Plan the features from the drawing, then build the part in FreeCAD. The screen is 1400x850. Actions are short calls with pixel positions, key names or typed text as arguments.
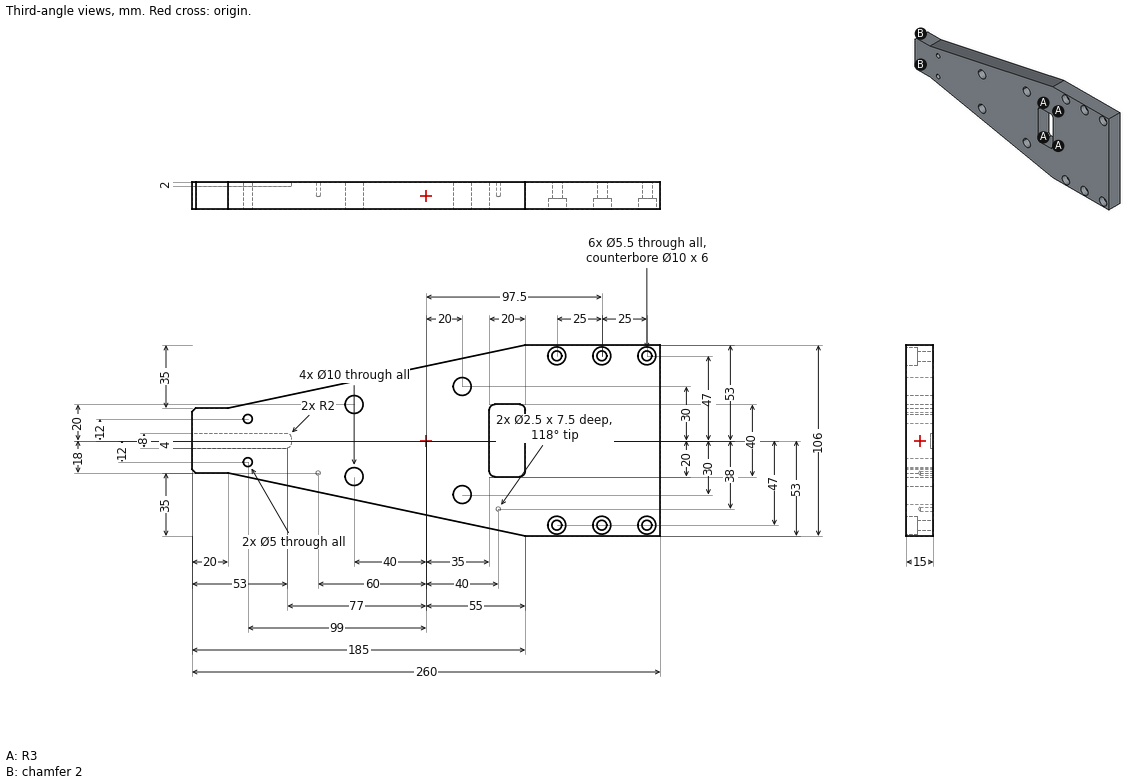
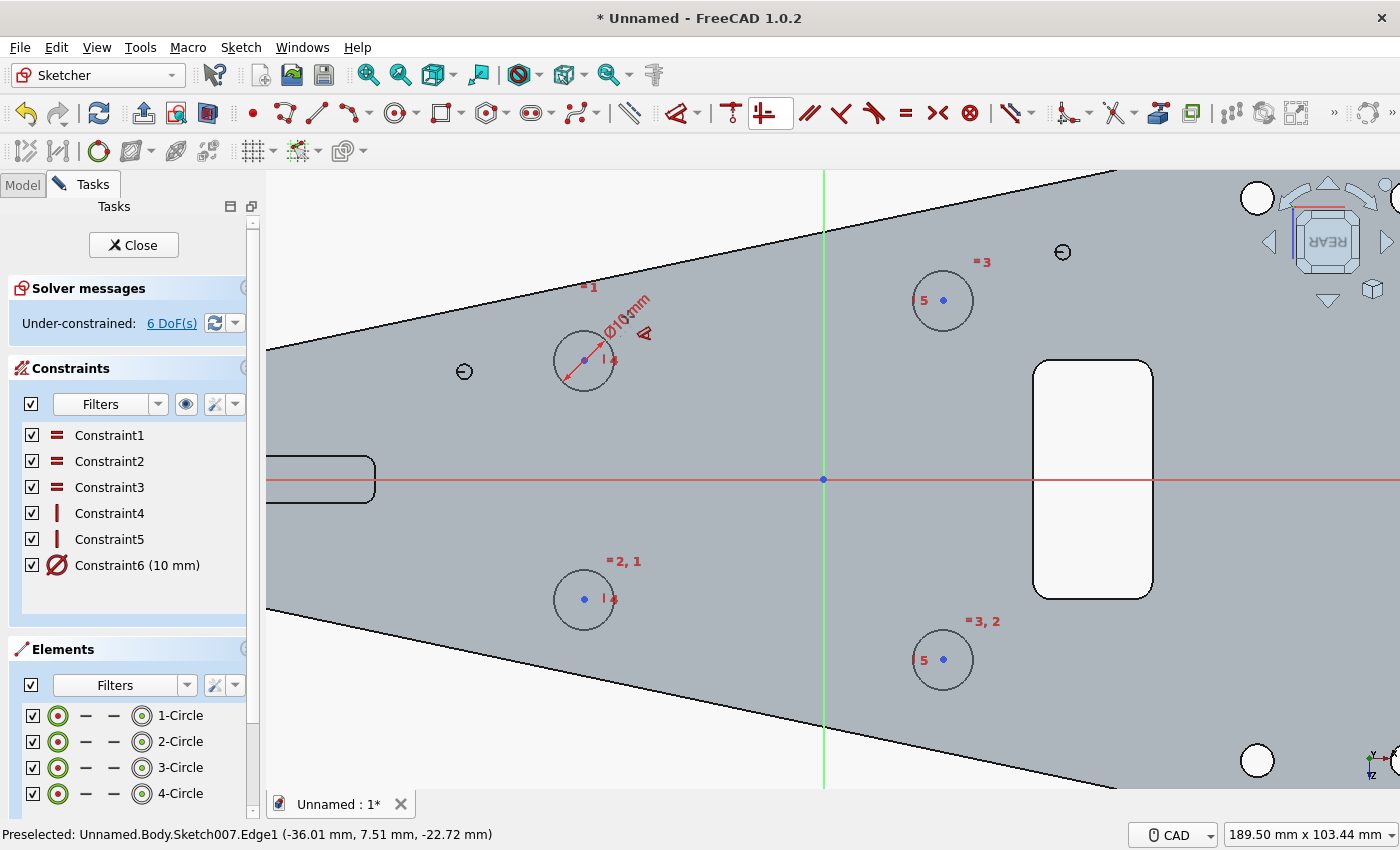
click(584, 361)
click(704, 327)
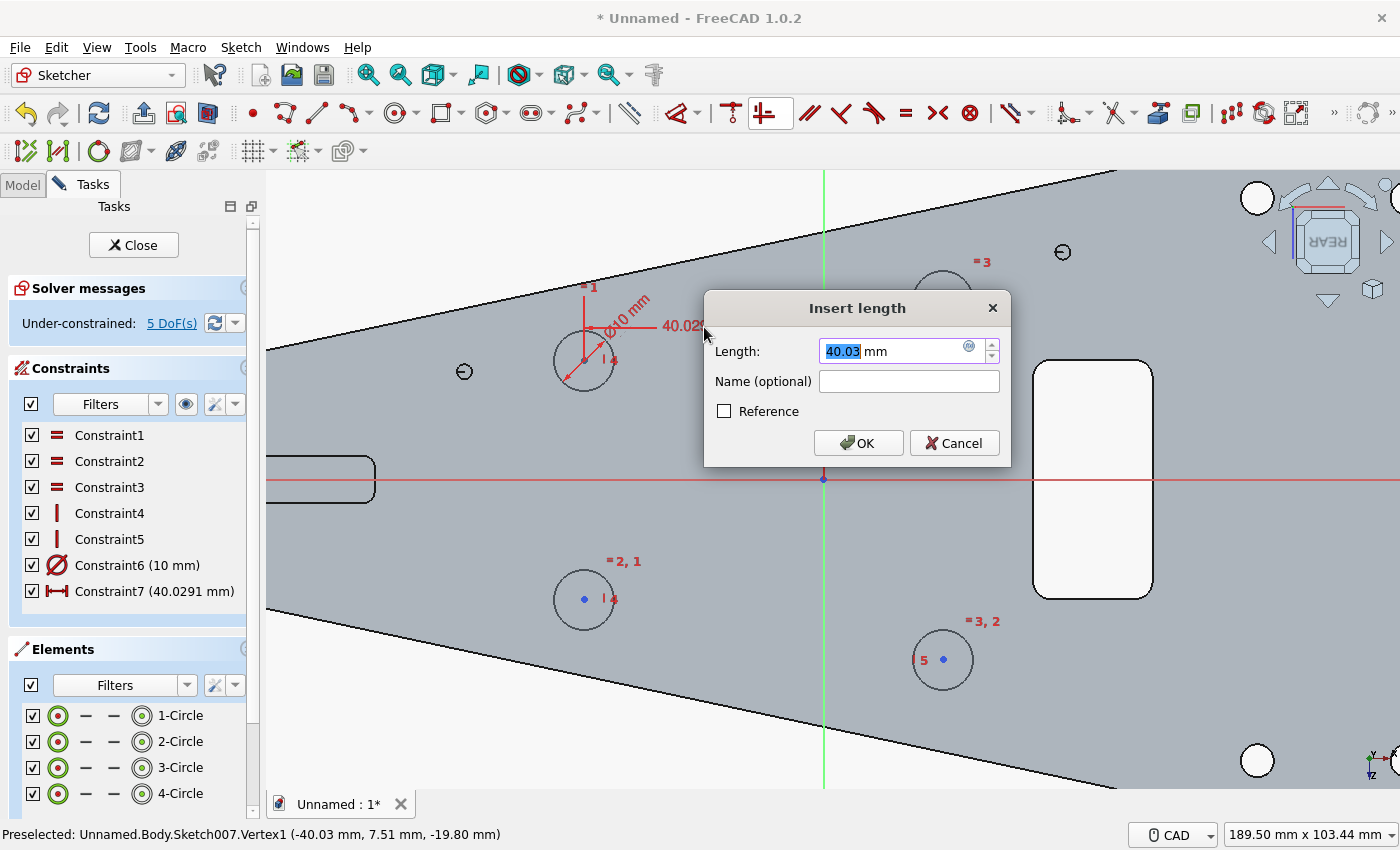
text(40)
key(Return)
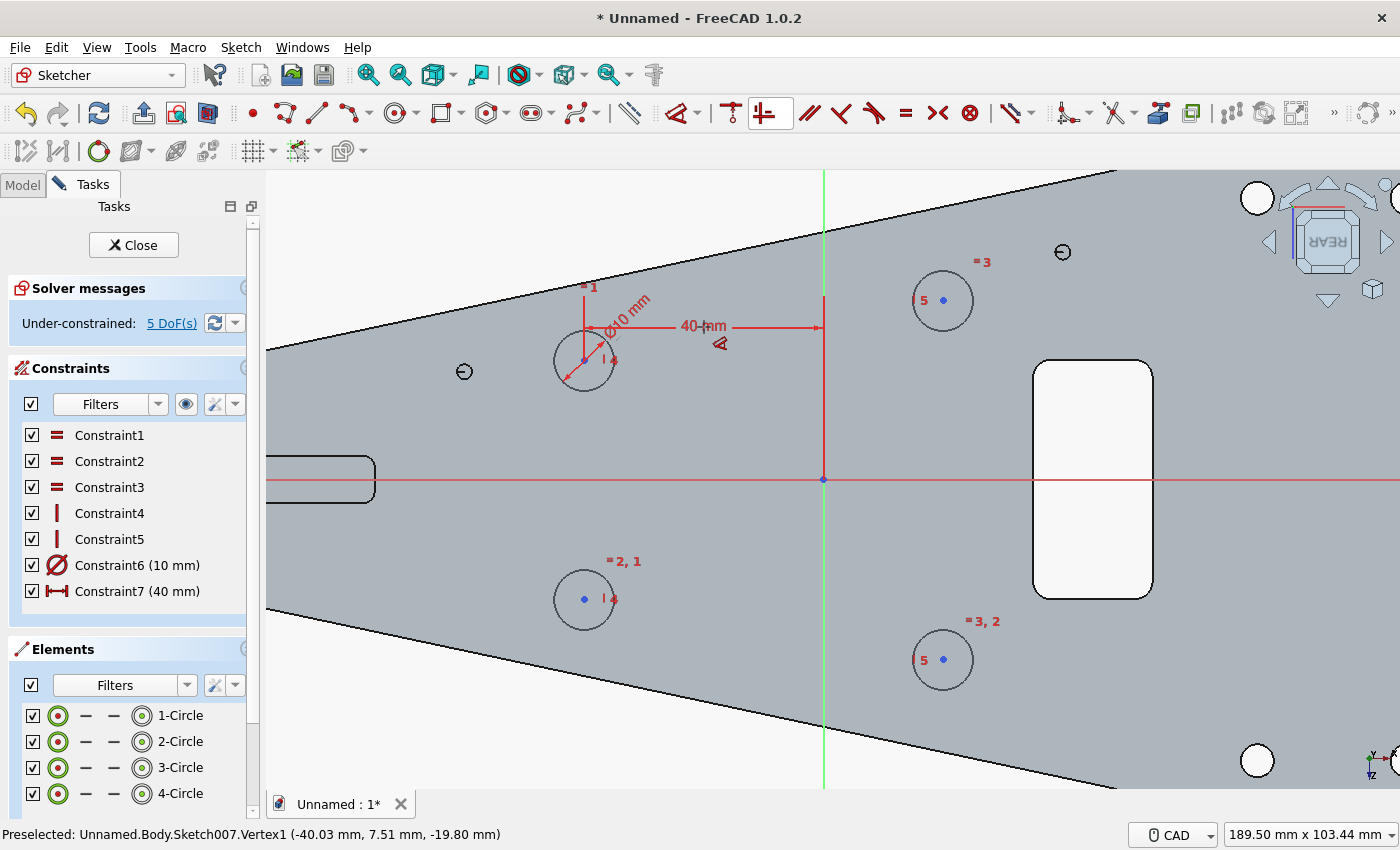
click(584, 361)
click(550, 420)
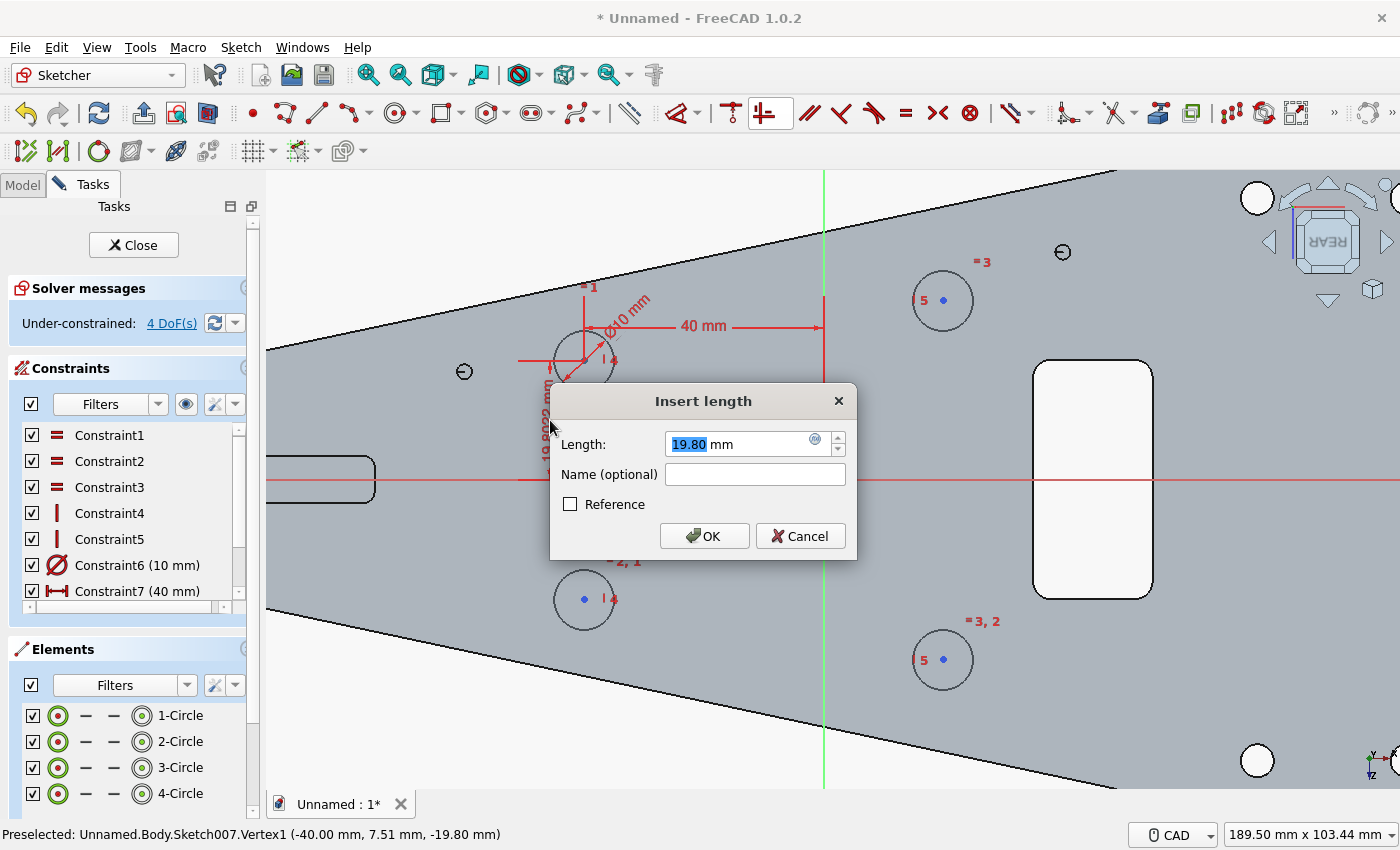
text(20)
key(Return)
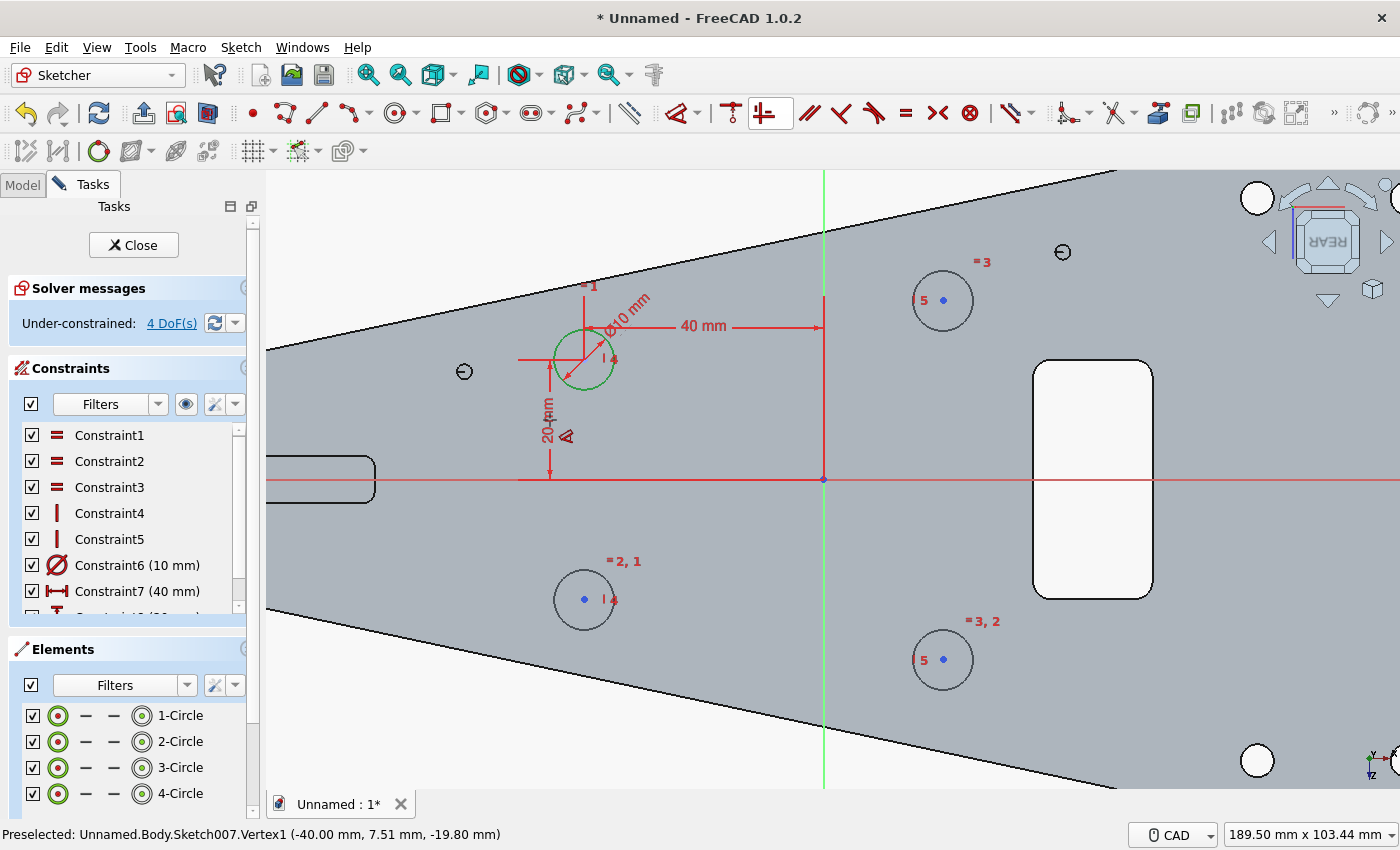
click(584, 600)
click(550, 540)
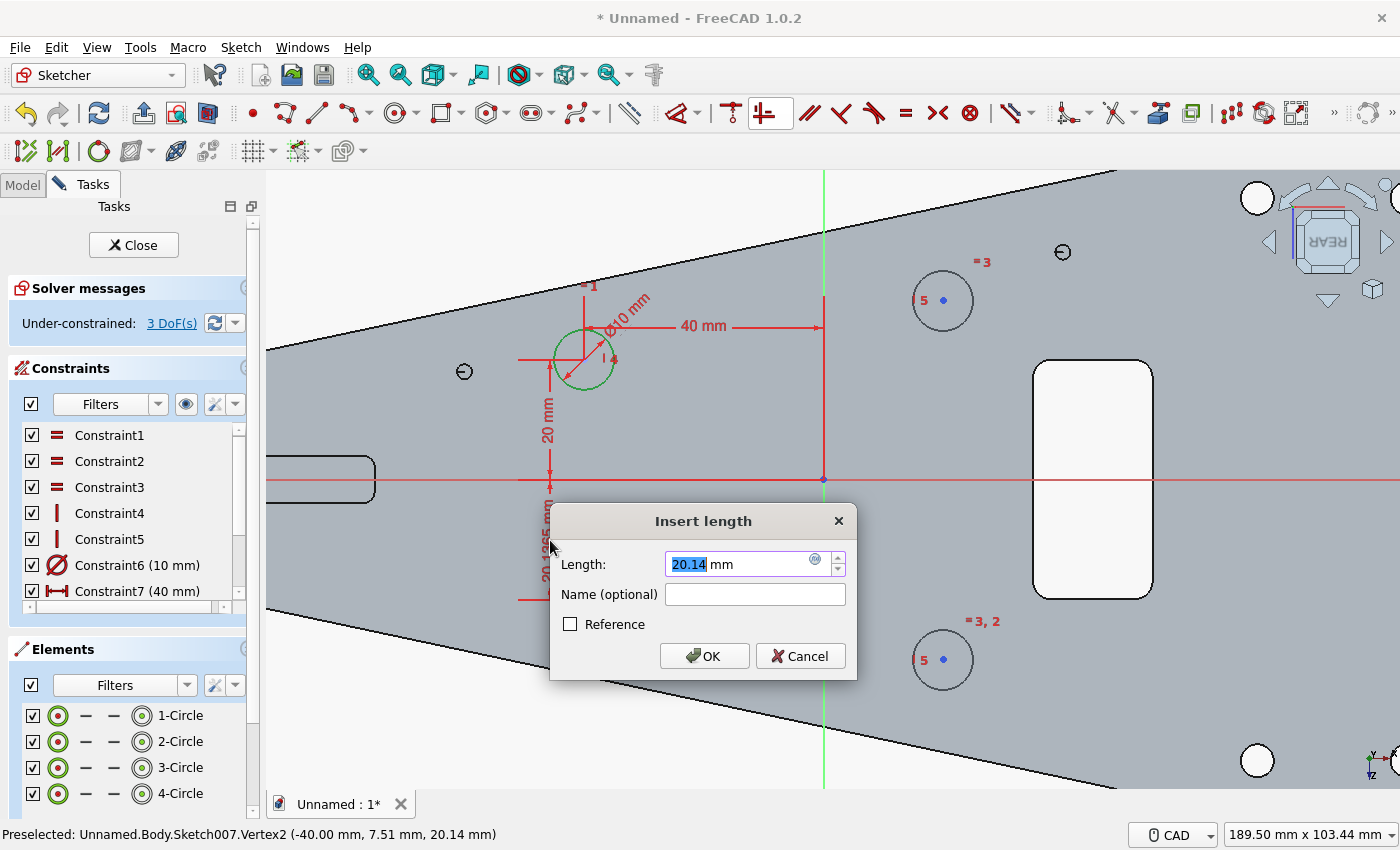
text(20)
key(Return)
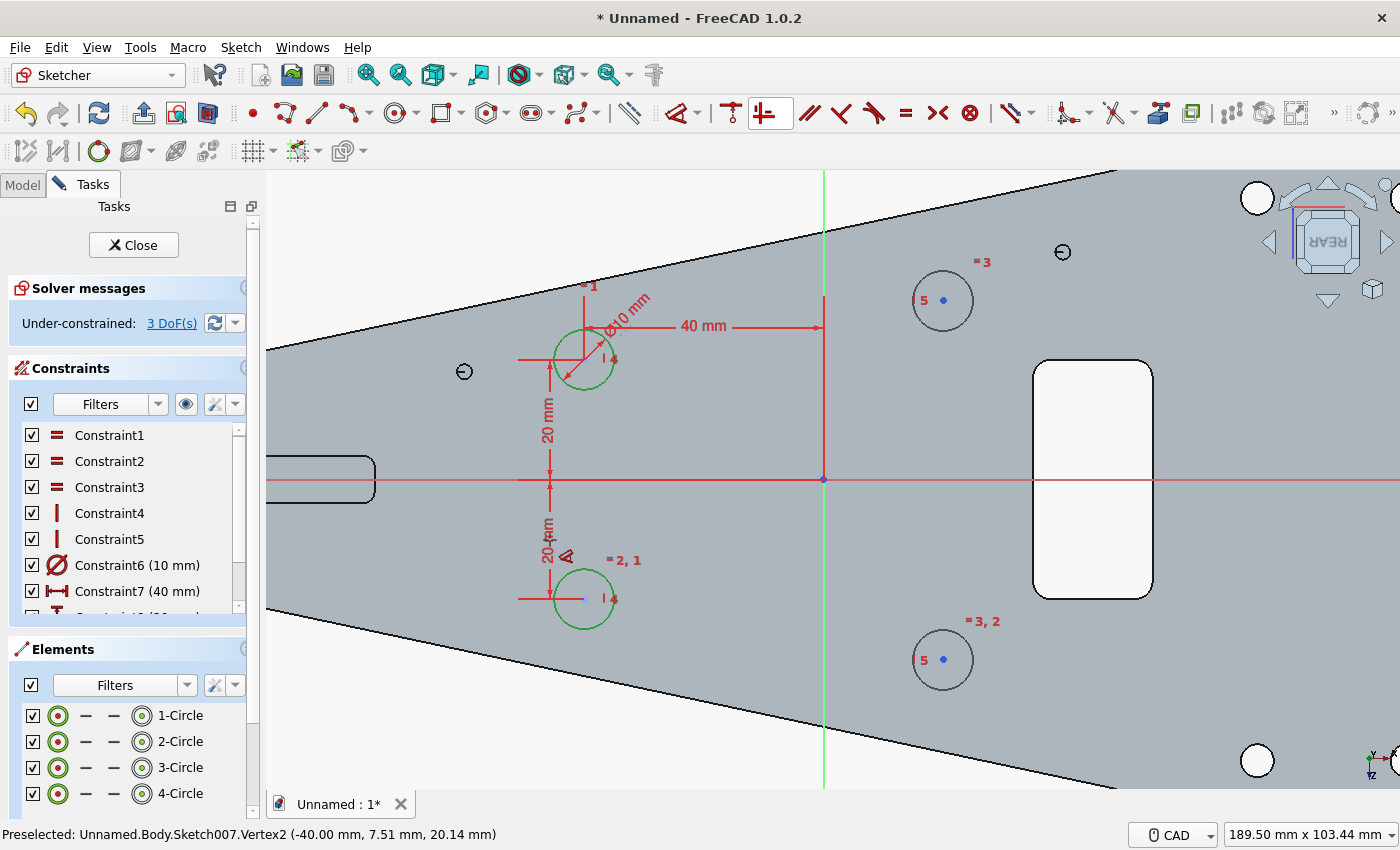
click(943, 660)
click(883, 694)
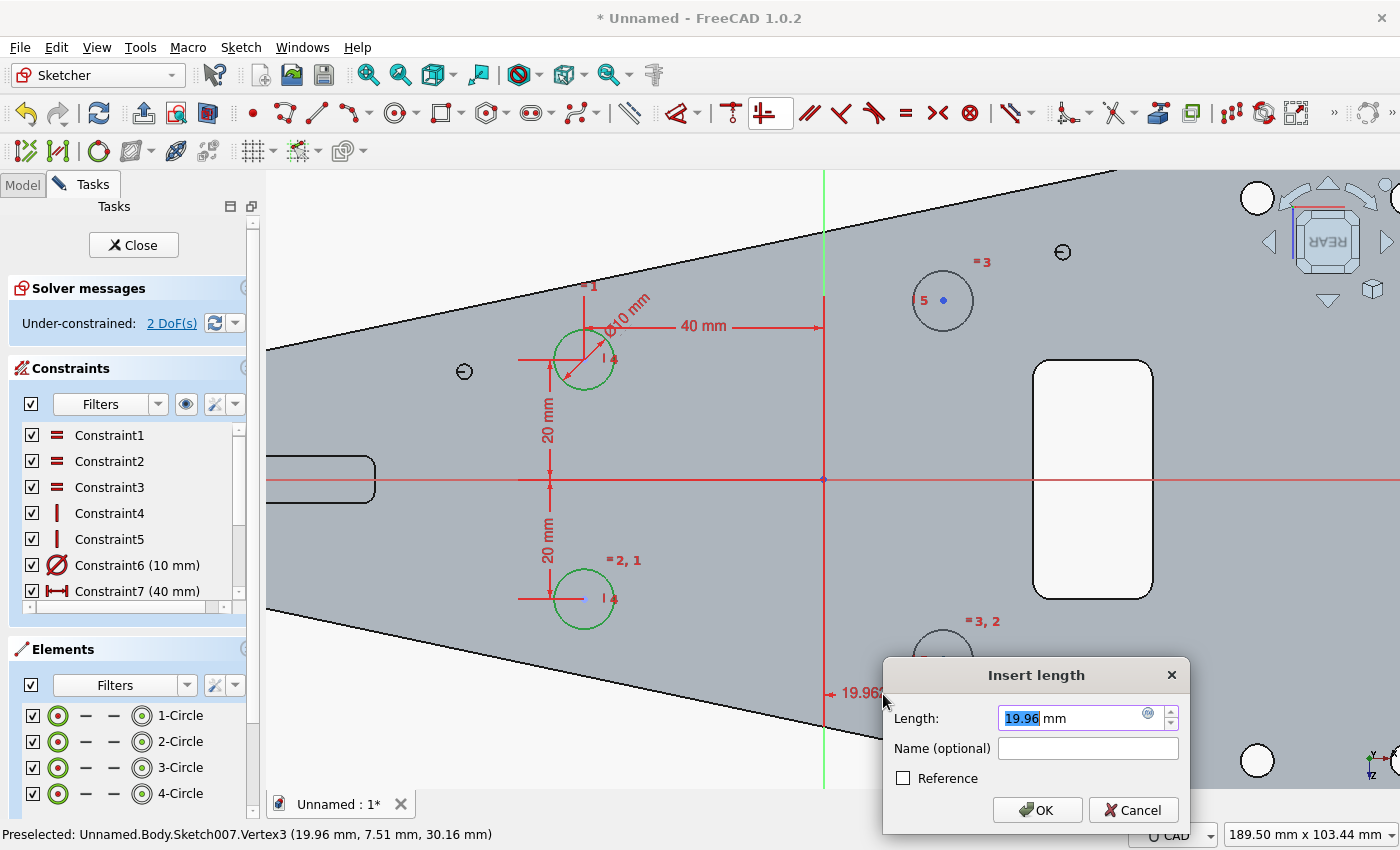
text(20)
key(Return)